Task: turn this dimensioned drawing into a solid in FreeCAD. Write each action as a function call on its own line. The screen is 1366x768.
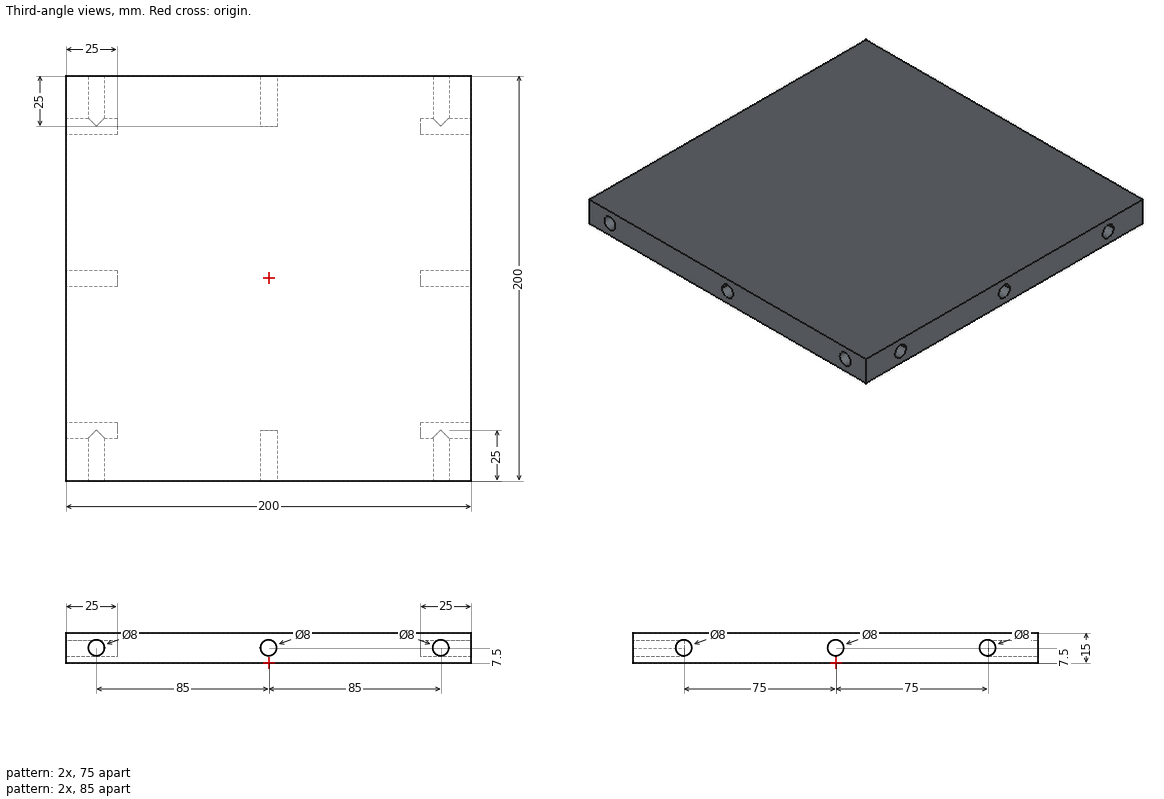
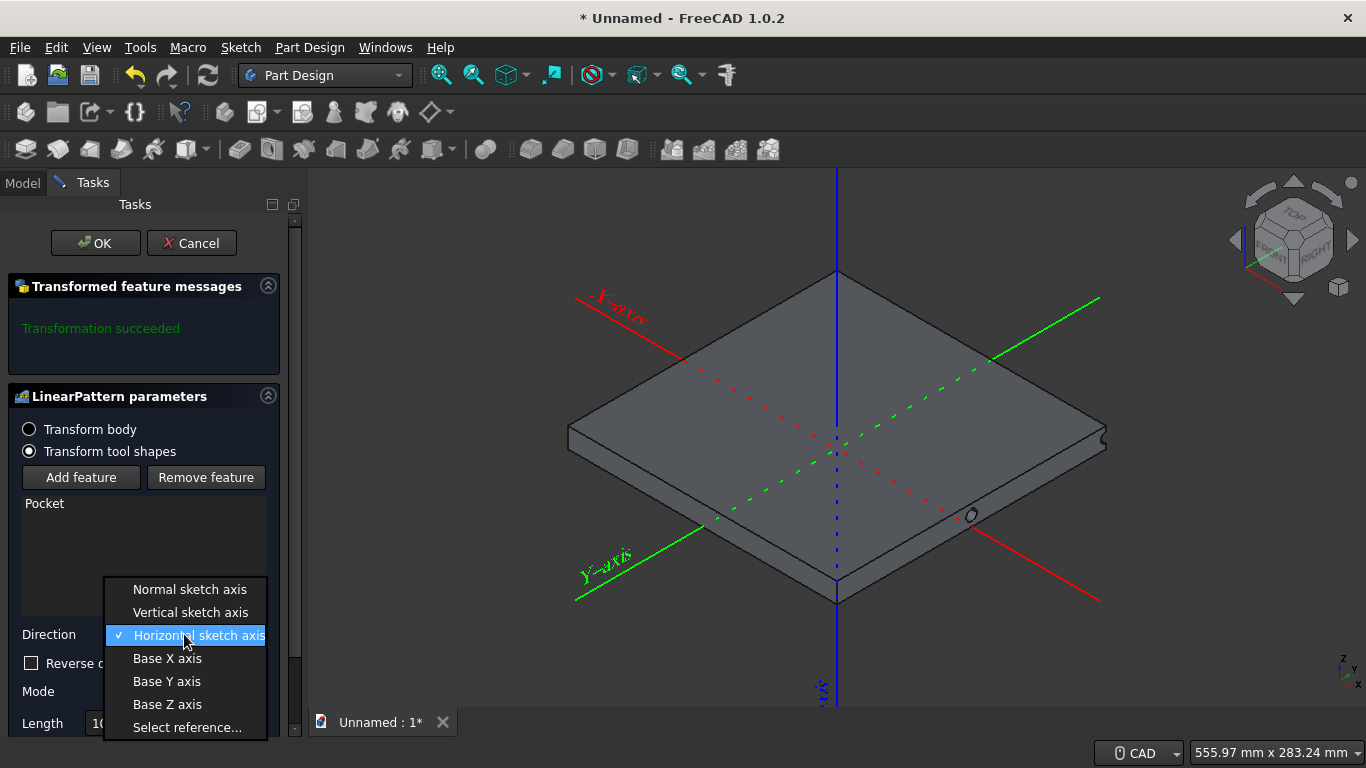
click(184, 682)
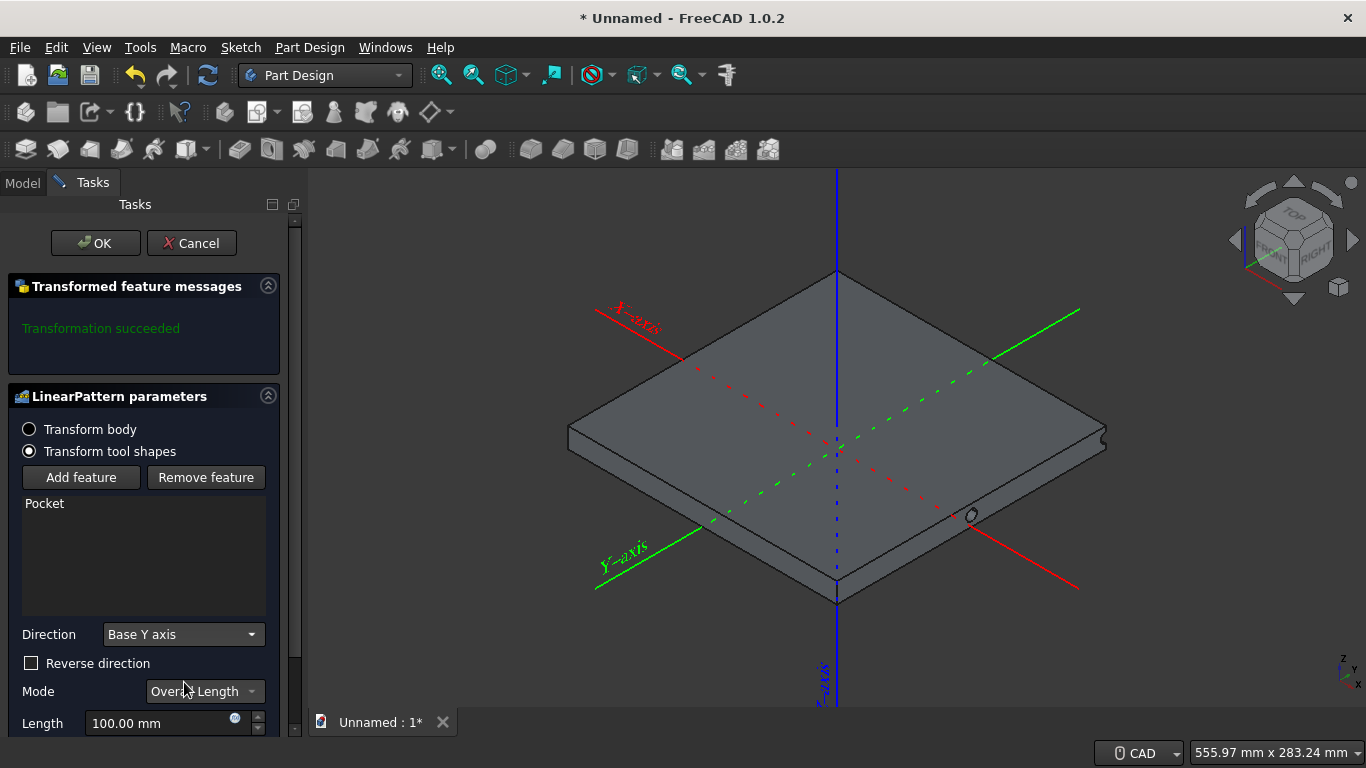
click(206, 692)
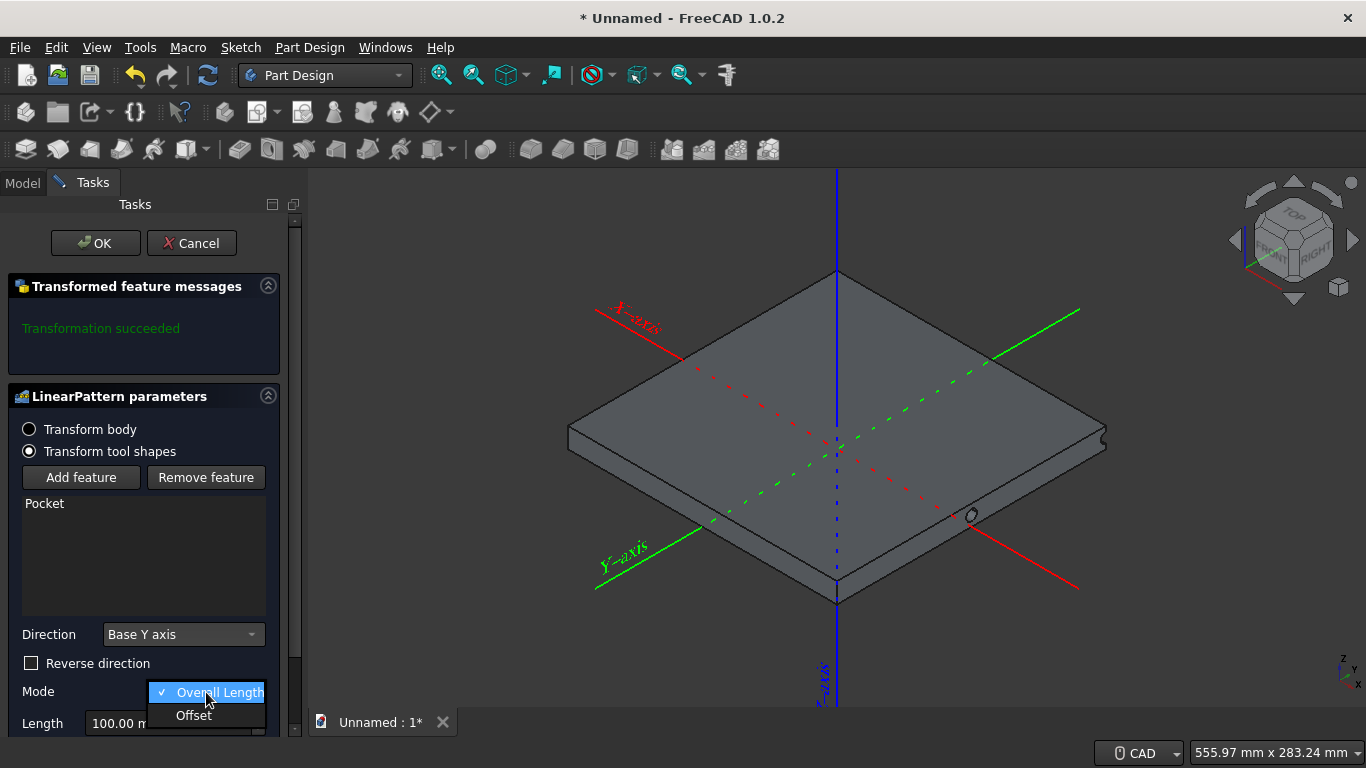
click(206, 716)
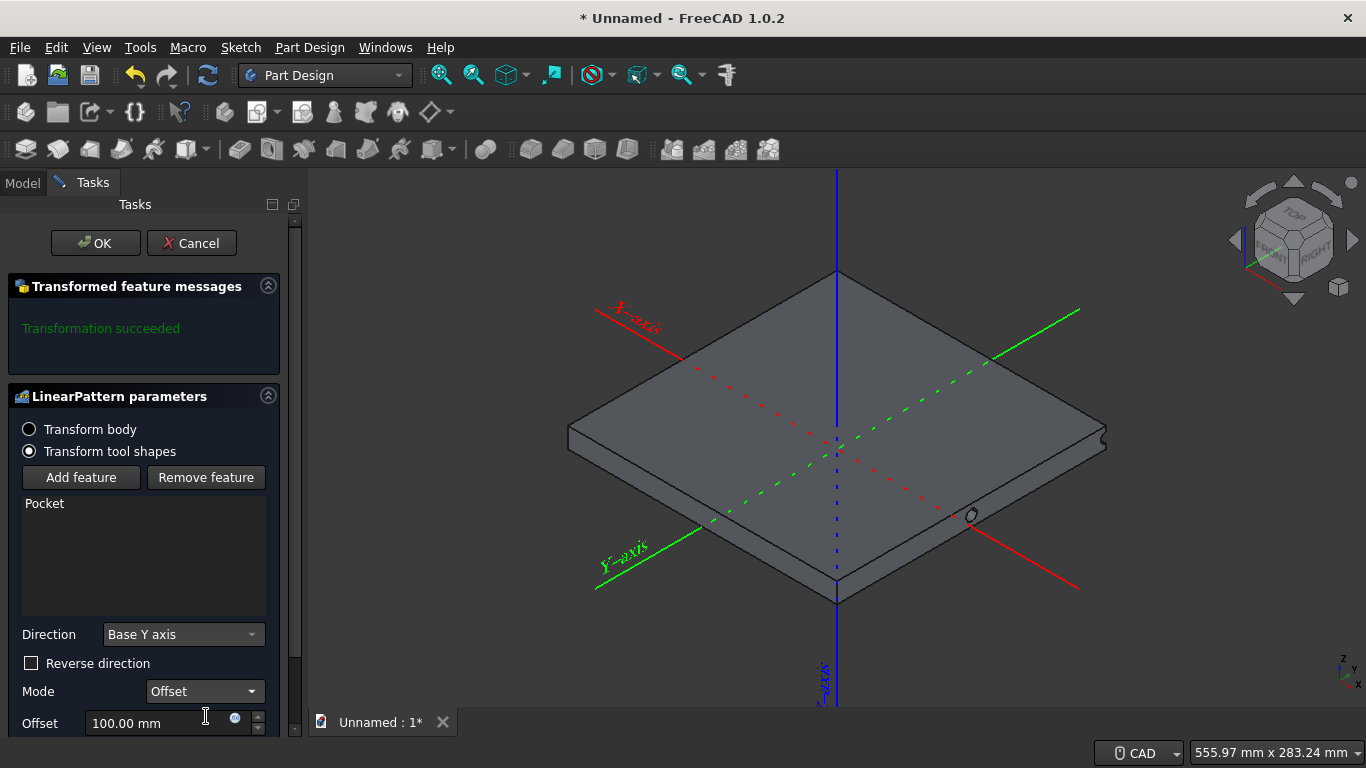
triple_click(168, 723)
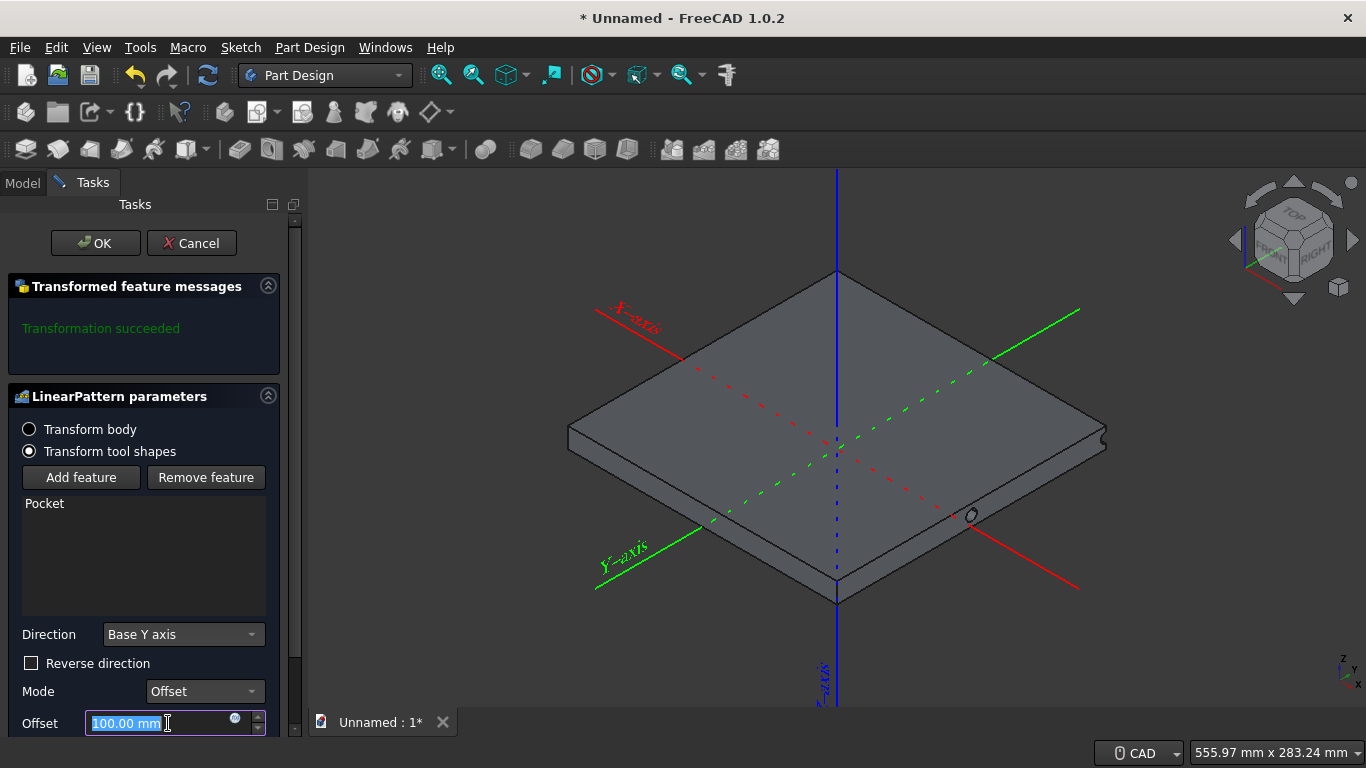
text(75)
key(Tab)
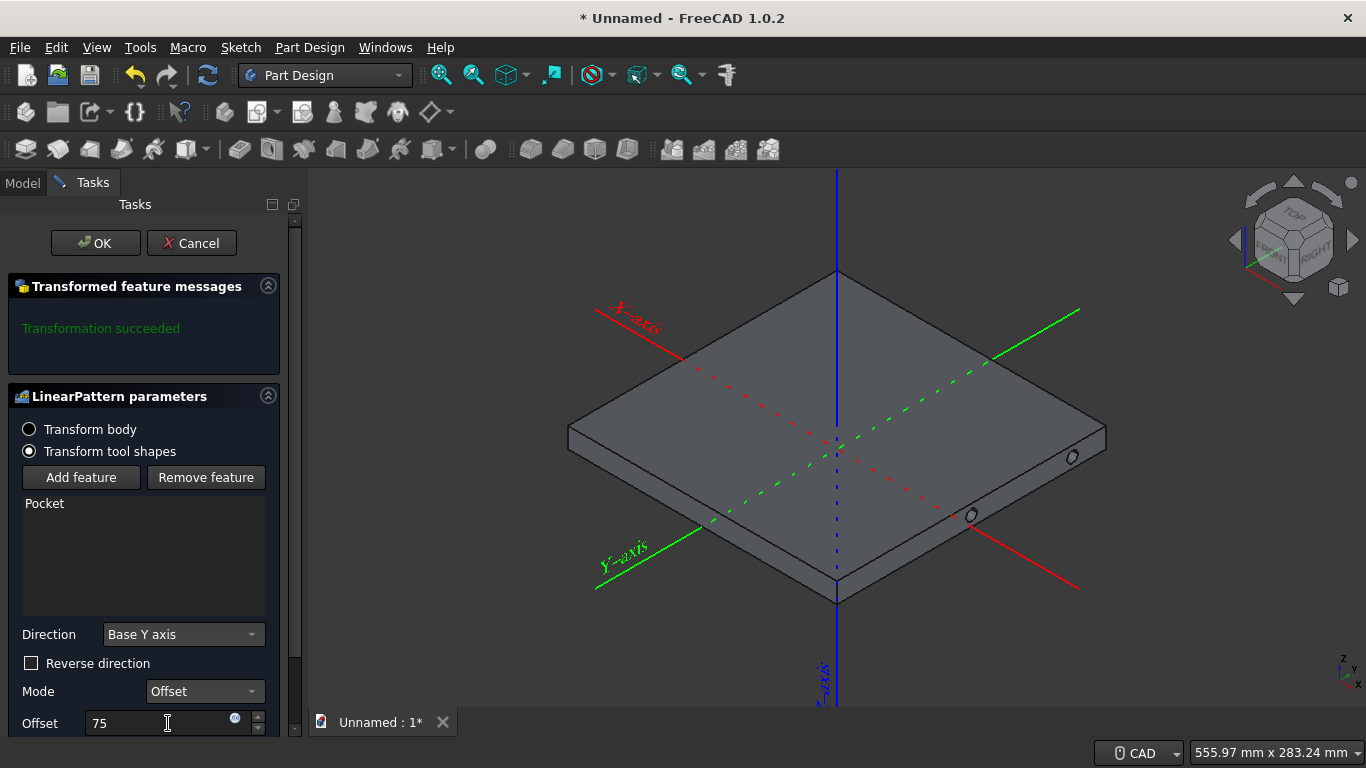
scroll(295, 475, down, 2)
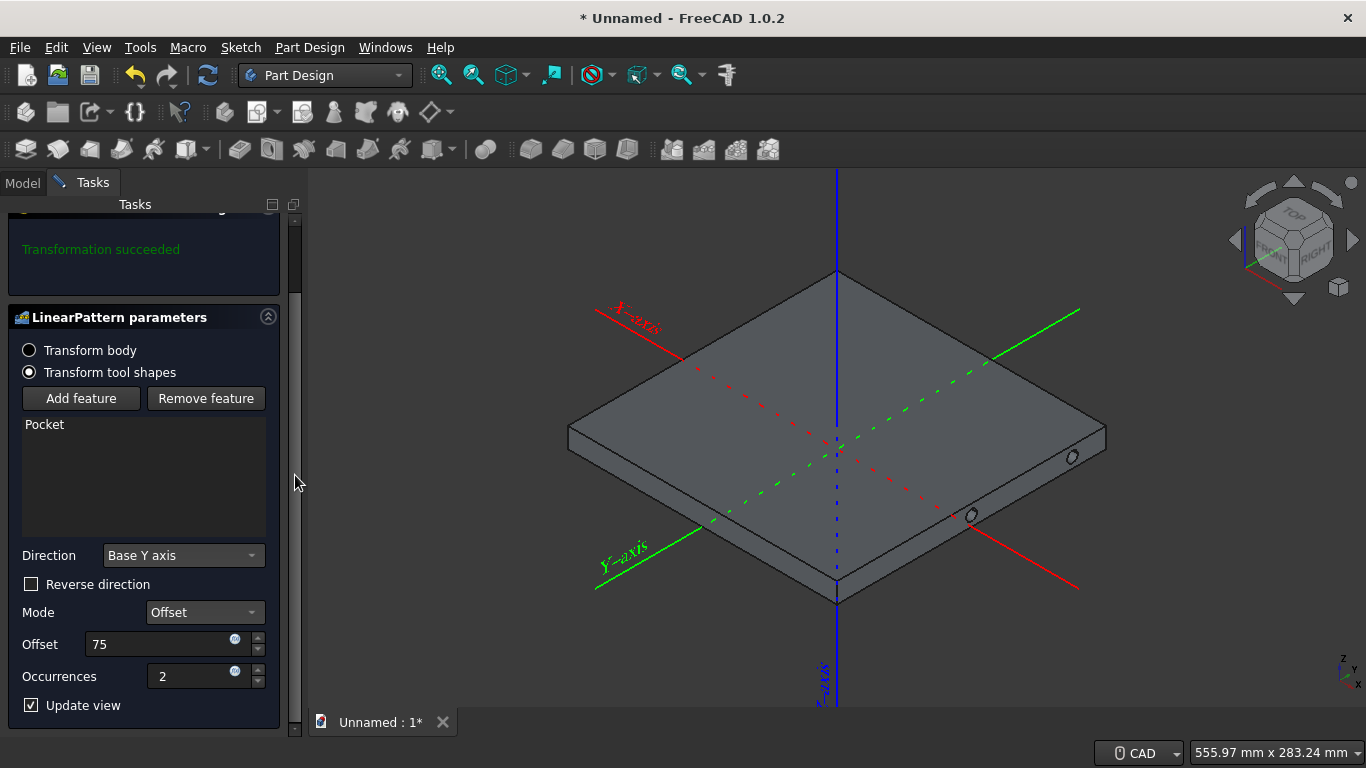
triple_click(198, 676)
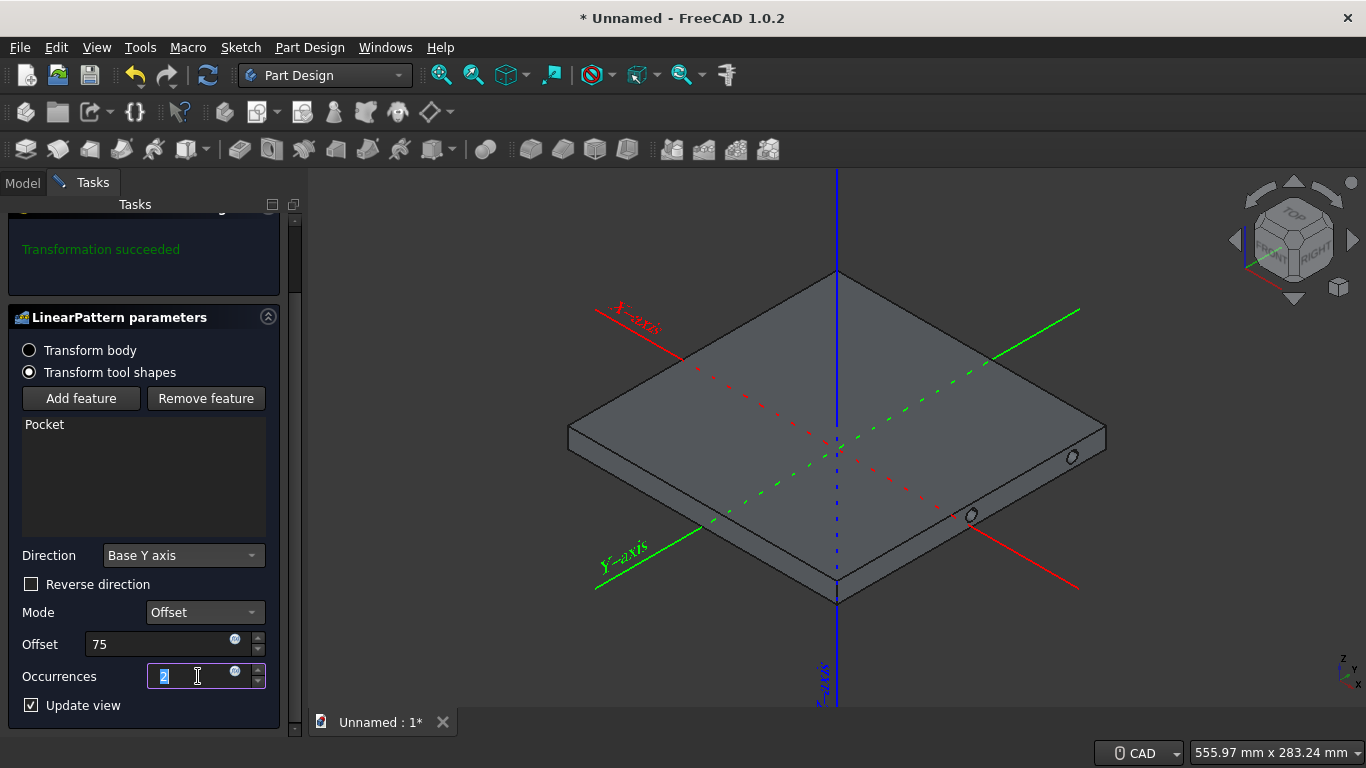
text(2)
key(Tab)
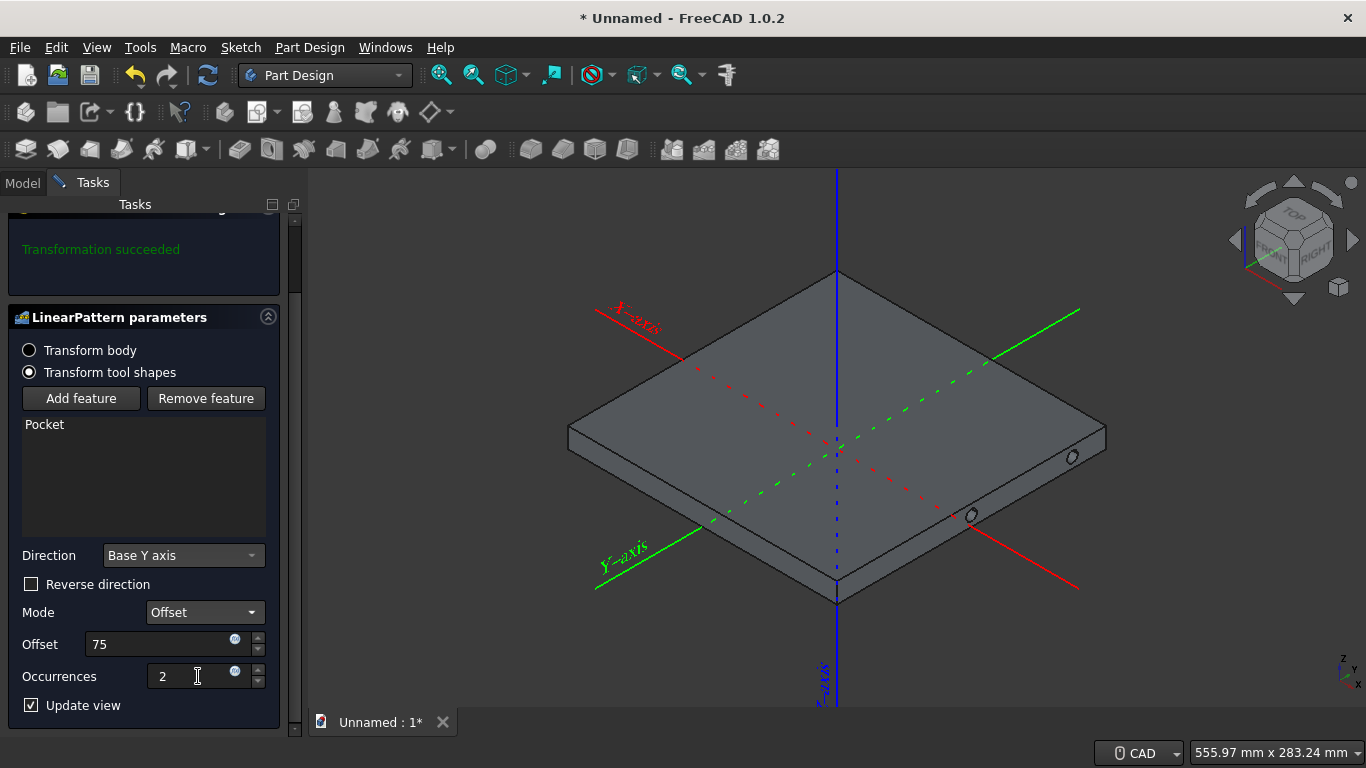
click(30, 584)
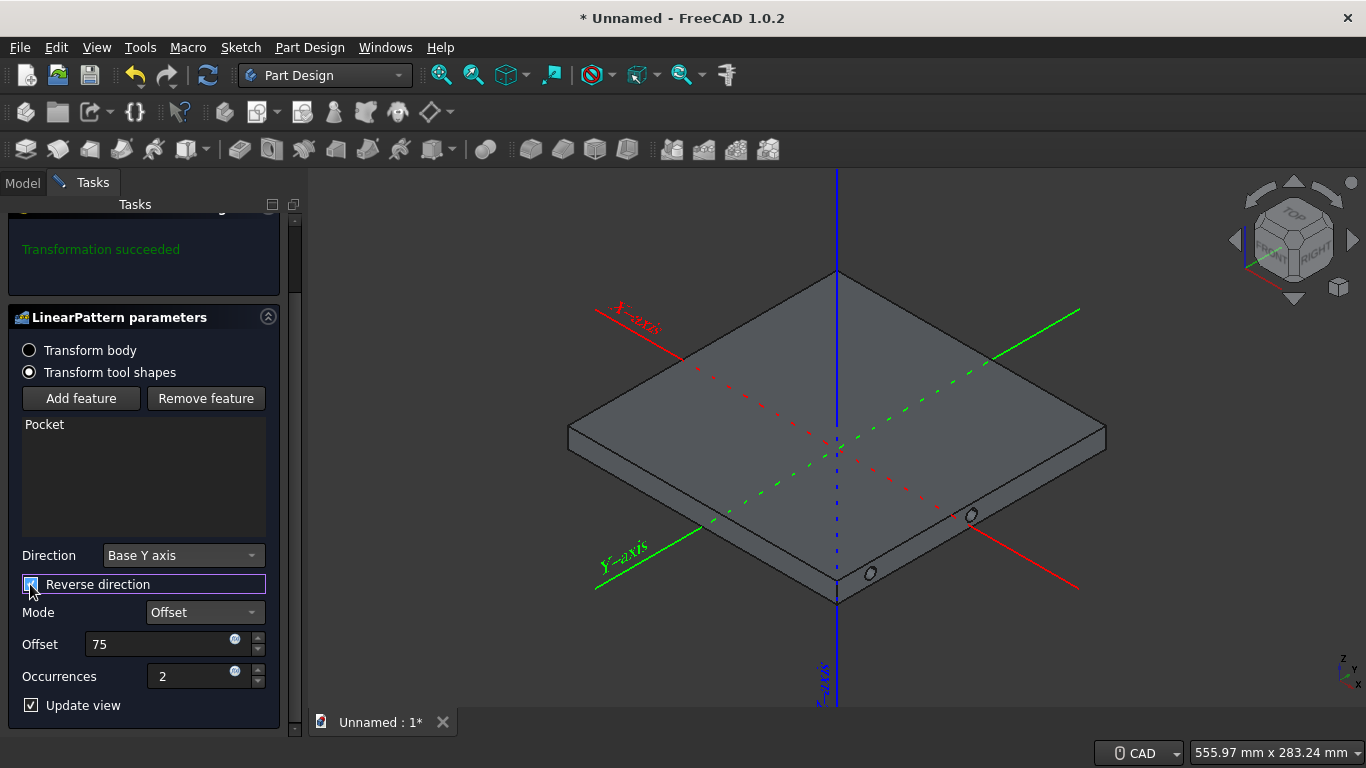
scroll(295, 475, up, 3)